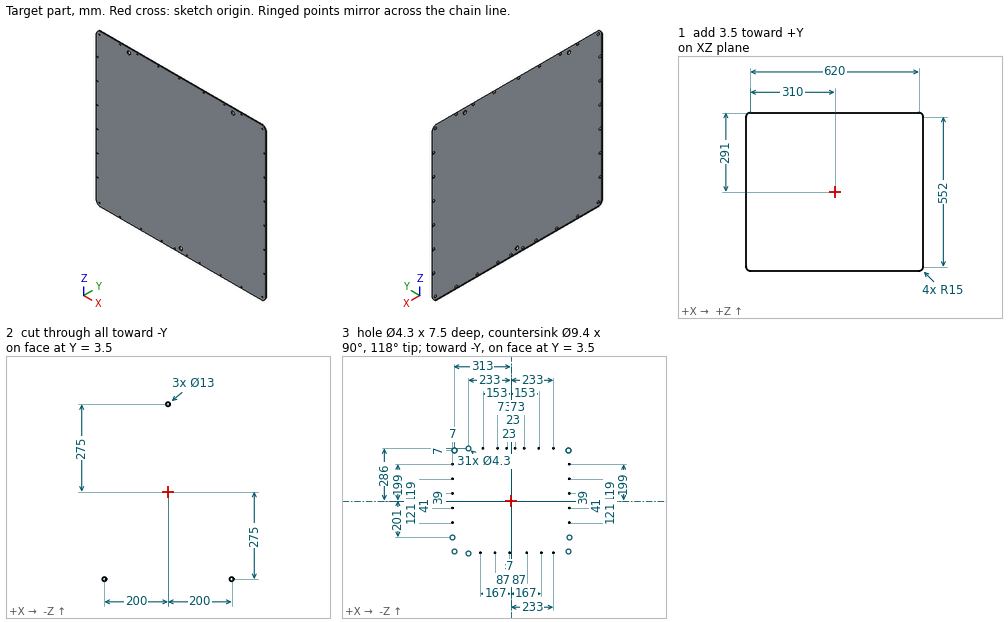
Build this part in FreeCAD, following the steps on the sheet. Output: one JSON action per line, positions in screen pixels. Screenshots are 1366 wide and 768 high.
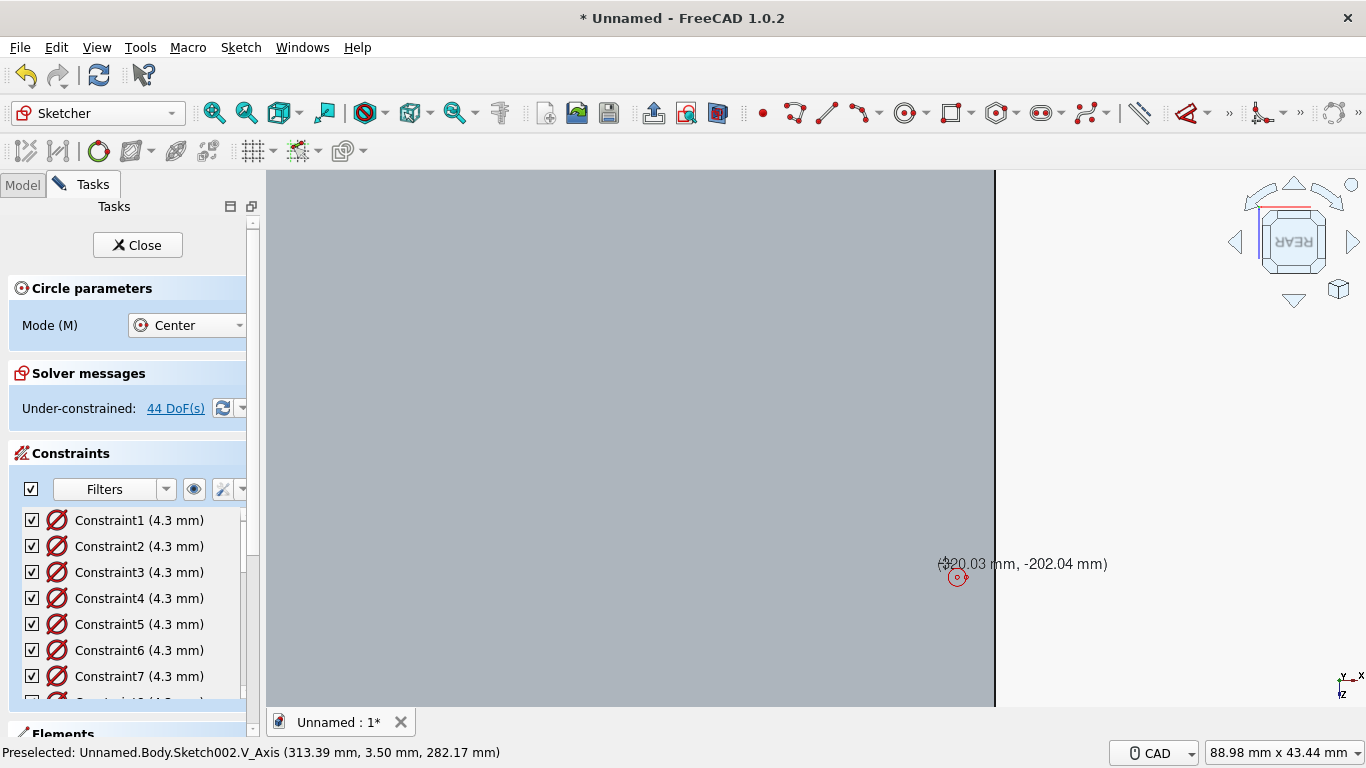
{"action": "scroll", "coordinate": [945, 563], "scroll_direction": "down", "scroll_amount": 15}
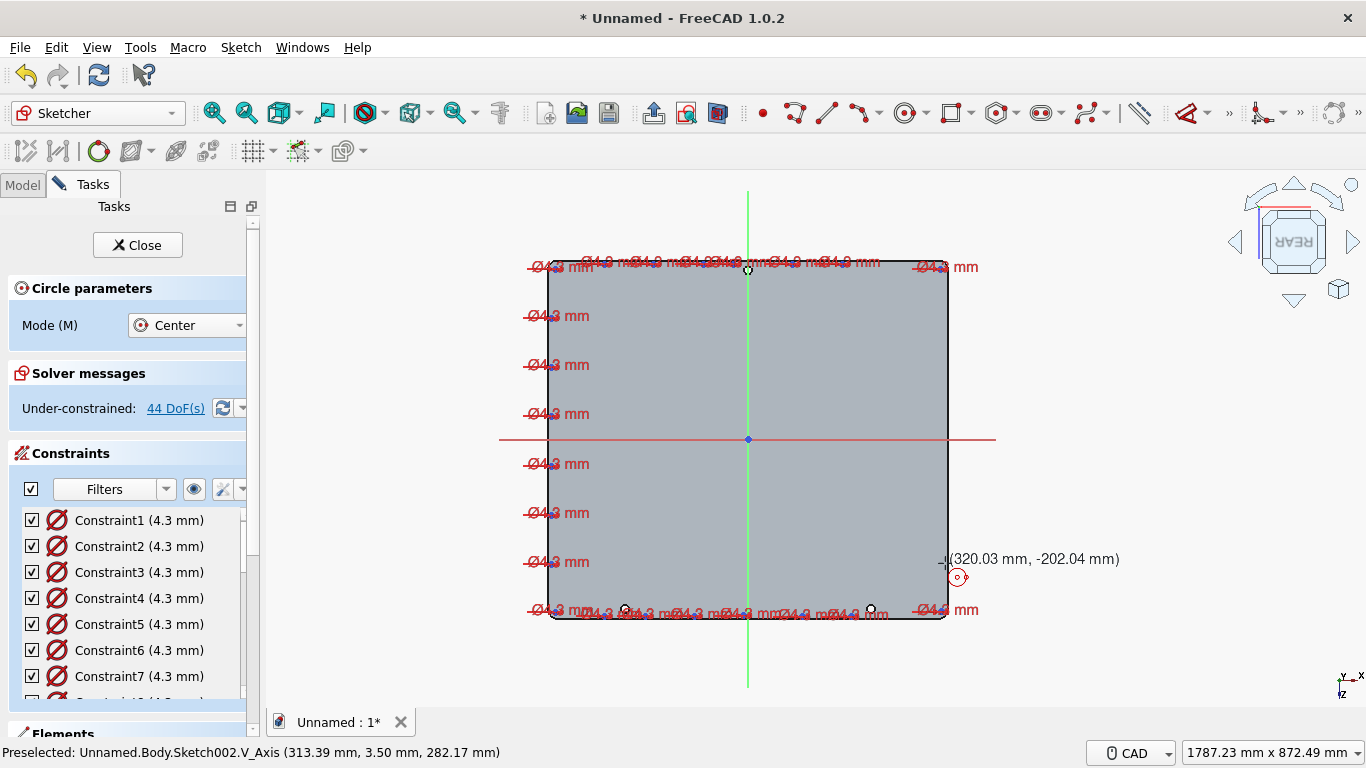
{"action": "left_click", "coordinate": [945, 563]}
{"action": "mouse_move", "coordinate": [946, 562]}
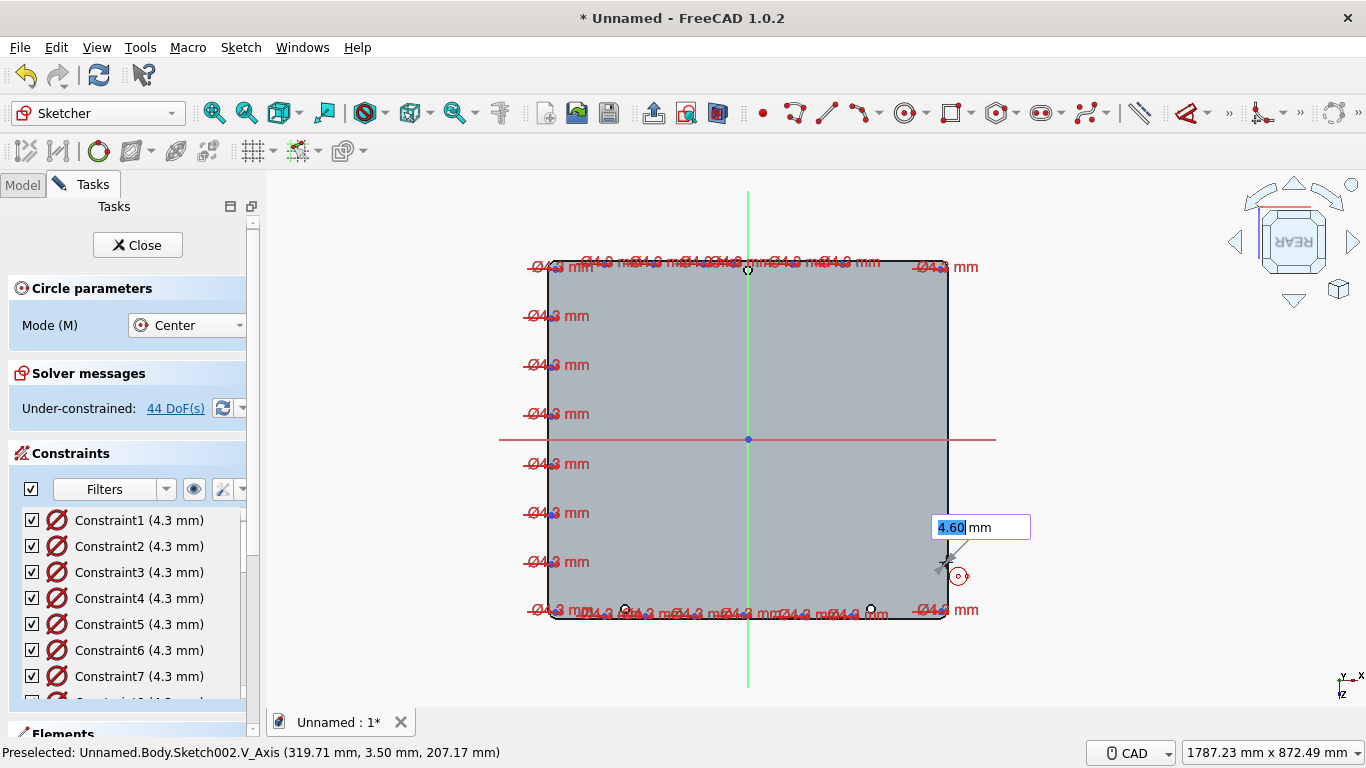
{"action": "type", "text": "4.3"}
{"action": "key", "text": "Return"}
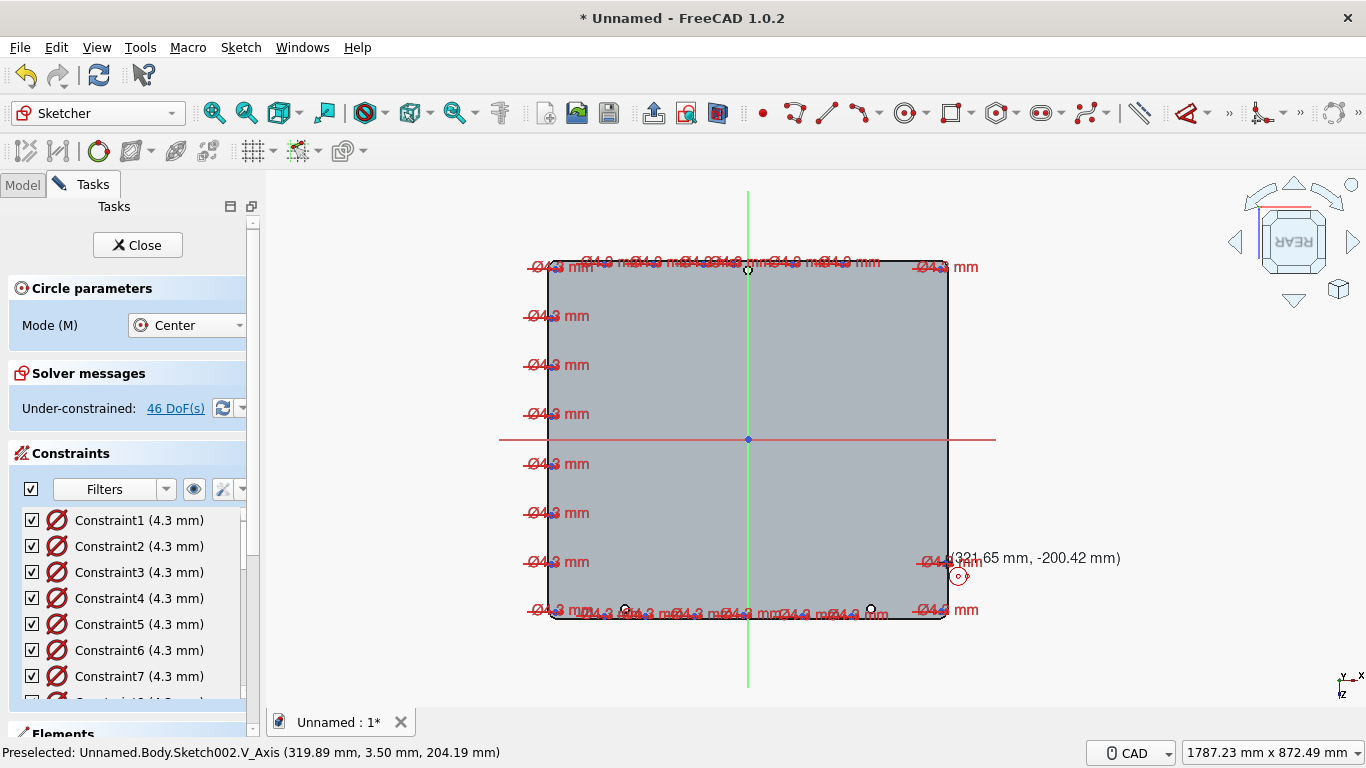
{"action": "scroll", "coordinate": [945, 514], "scroll_direction": "up", "scroll_amount": 15}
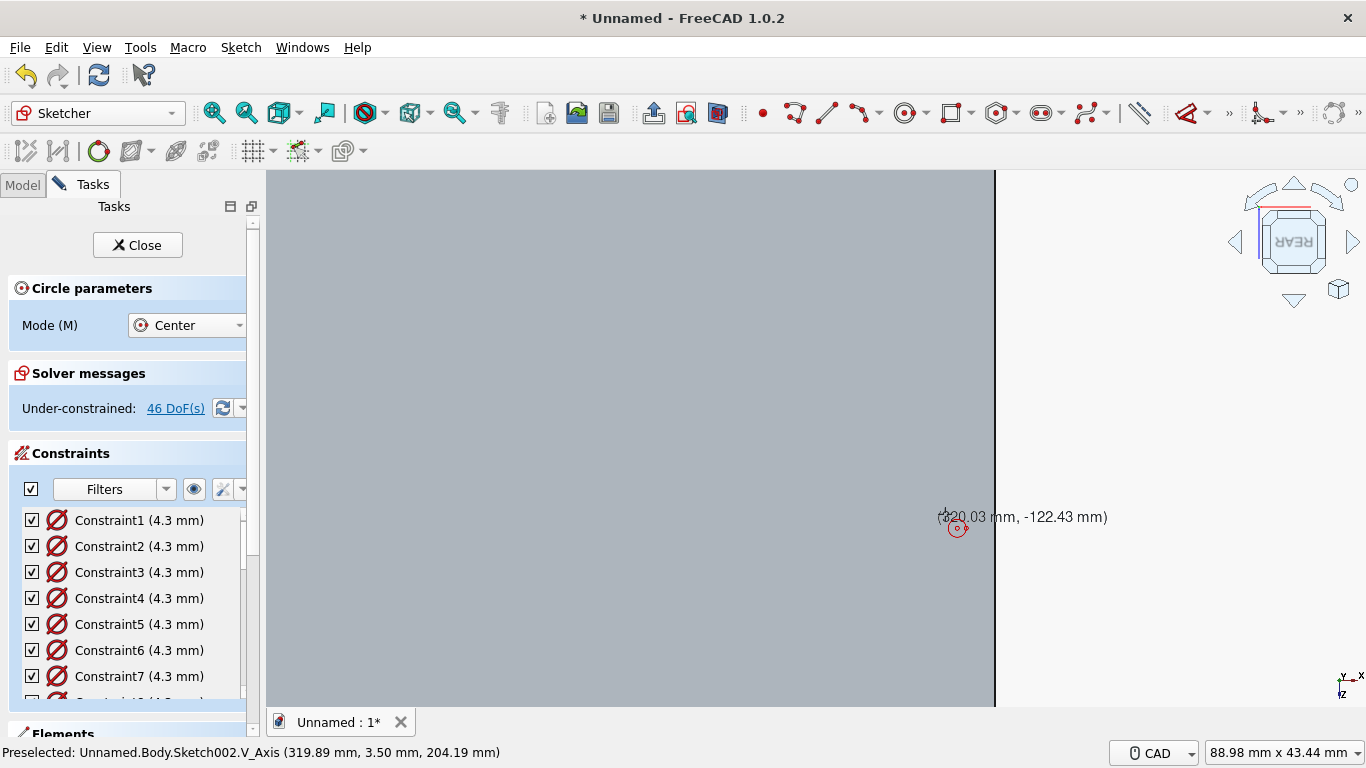
{"action": "scroll", "coordinate": [945, 513], "scroll_direction": "down", "scroll_amount": 15}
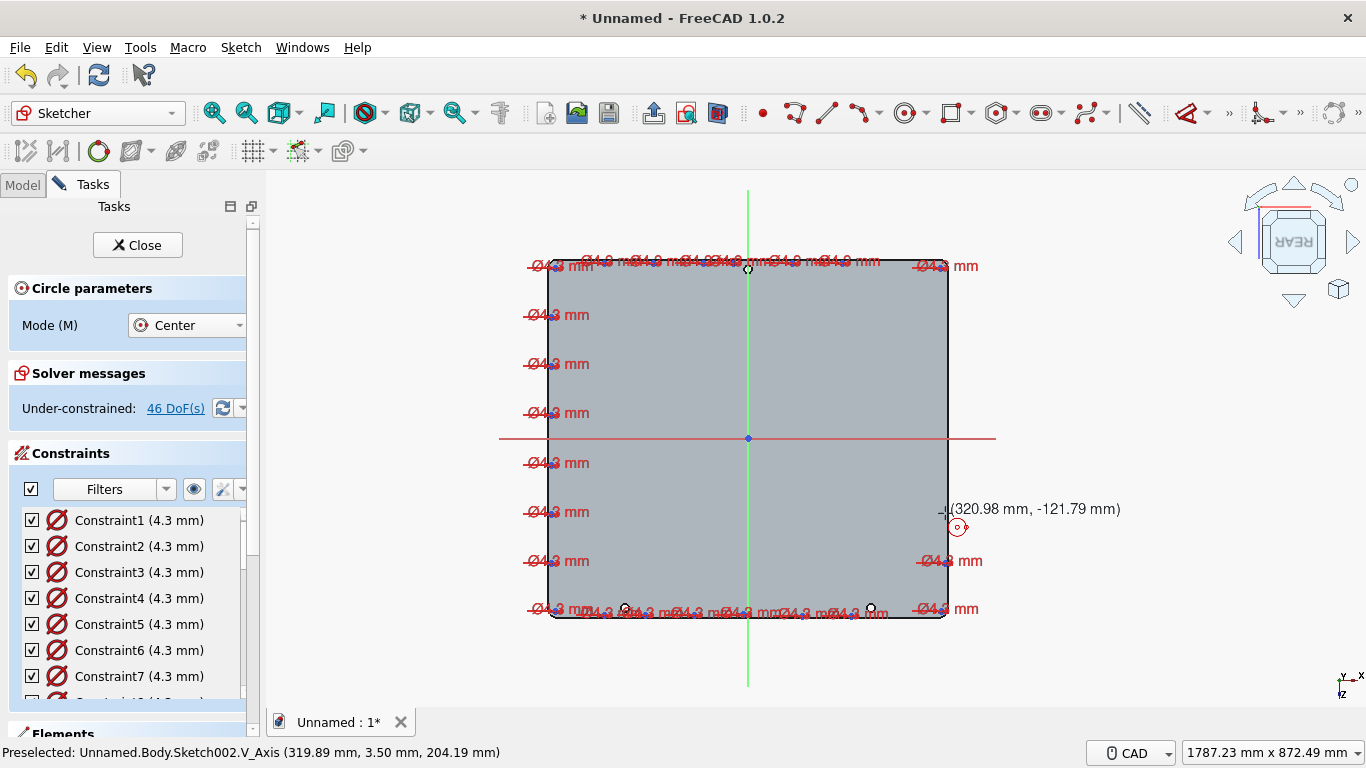
{"action": "left_click", "coordinate": [945, 513]}
{"action": "mouse_move", "coordinate": [946, 512]}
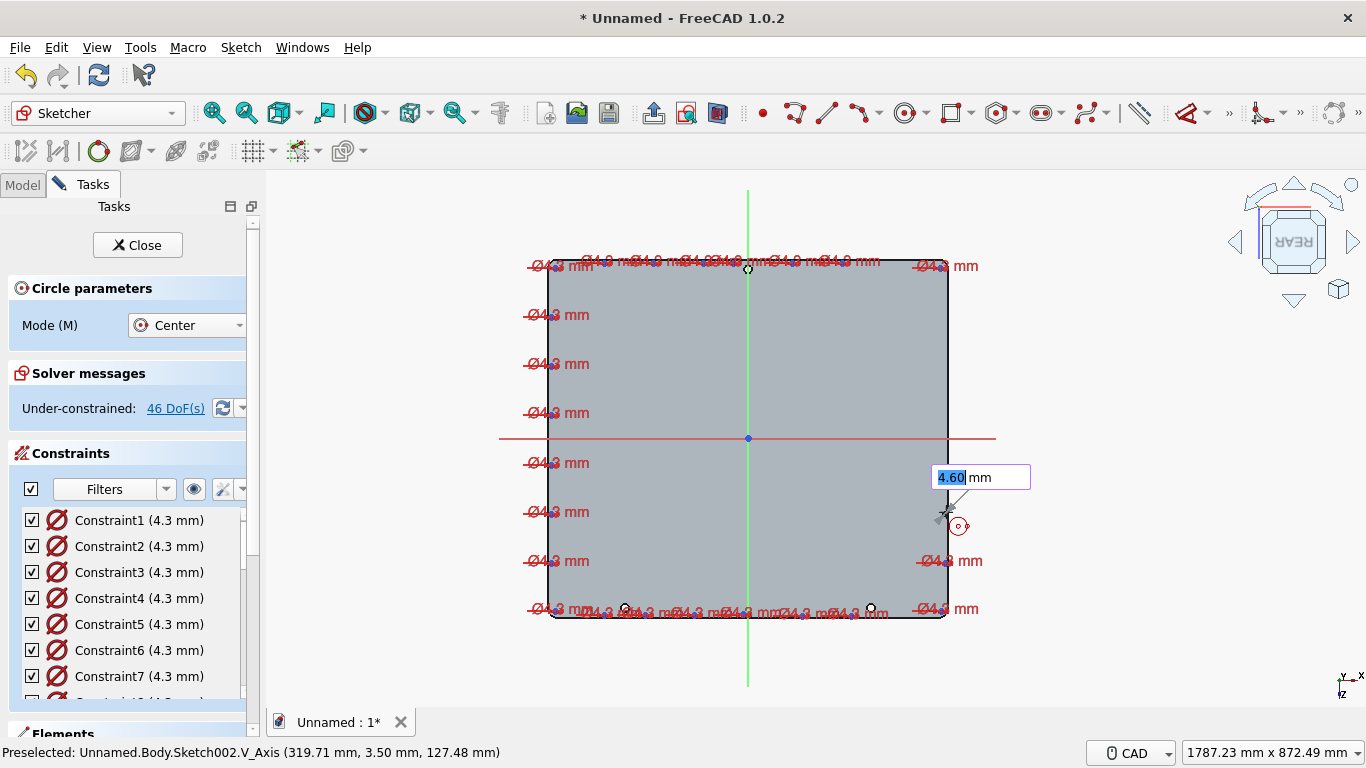
{"action": "type", "text": "4.3"}
{"action": "key", "text": "Return"}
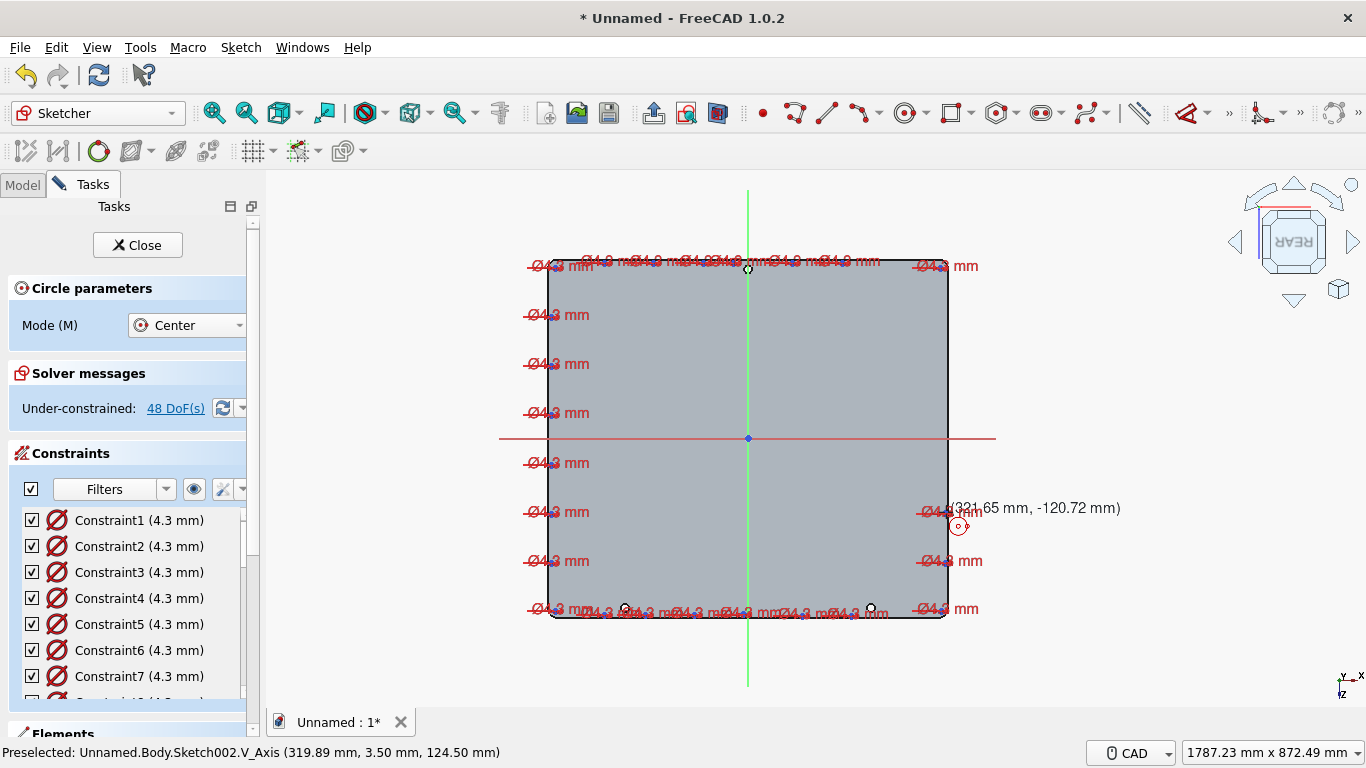
{"action": "scroll", "coordinate": [945, 464], "scroll_direction": "up", "scroll_amount": 15}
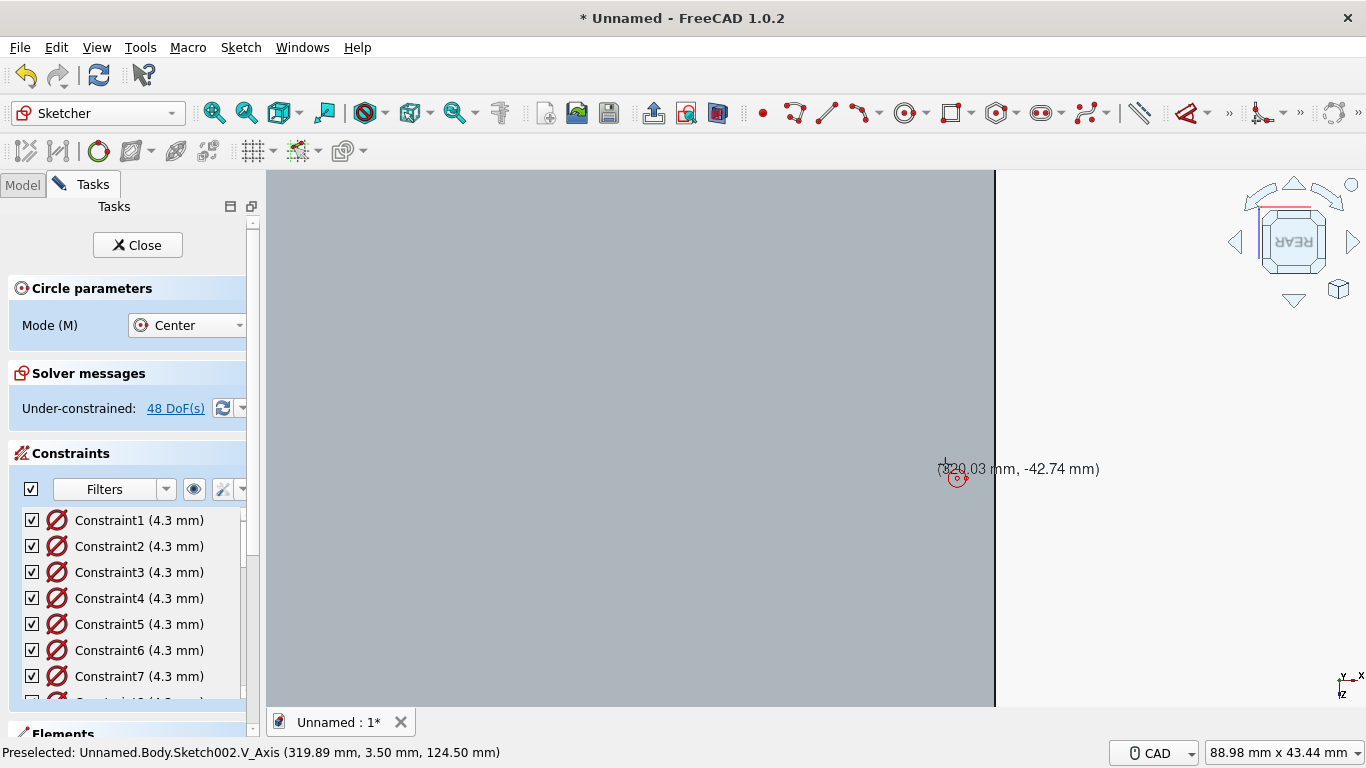
{"action": "scroll", "coordinate": [945, 464], "scroll_direction": "down", "scroll_amount": 15}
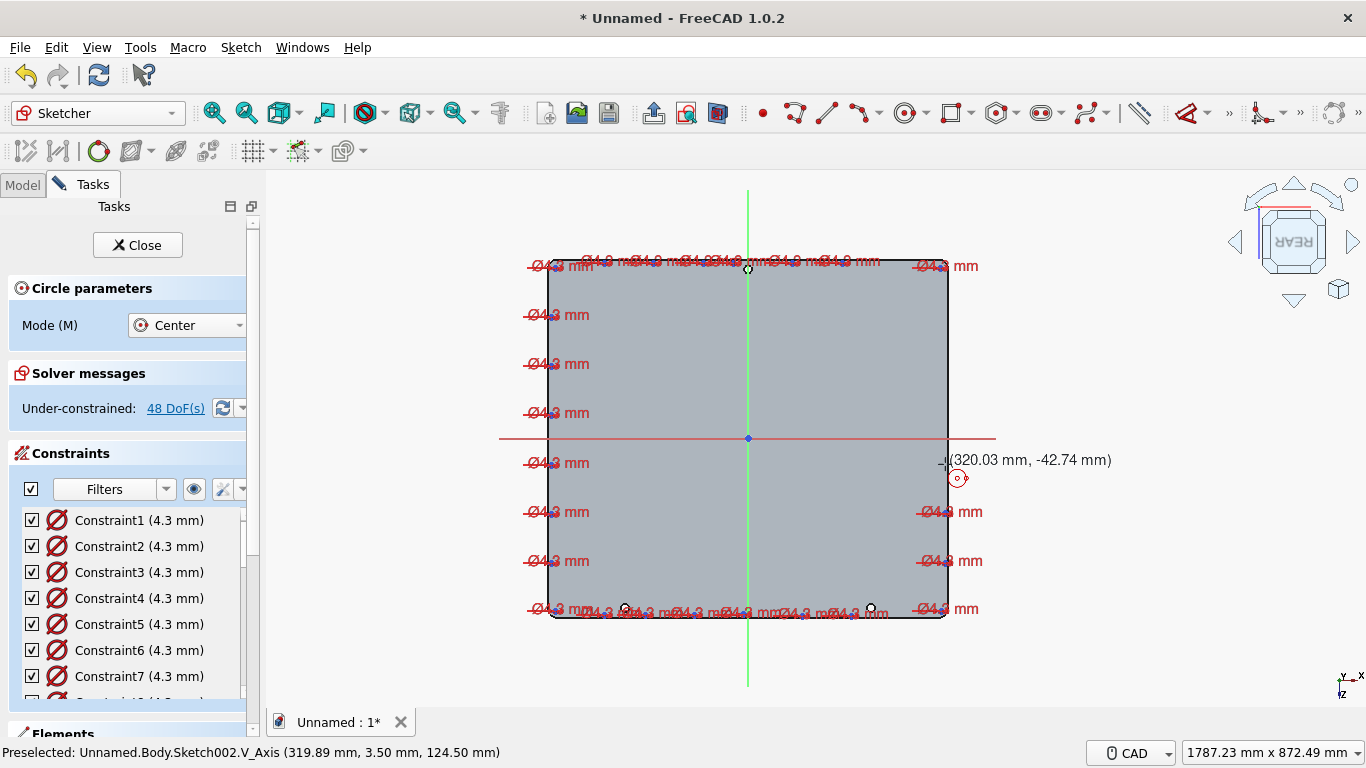
{"action": "left_click", "coordinate": [945, 464]}
{"action": "mouse_move", "coordinate": [946, 463]}